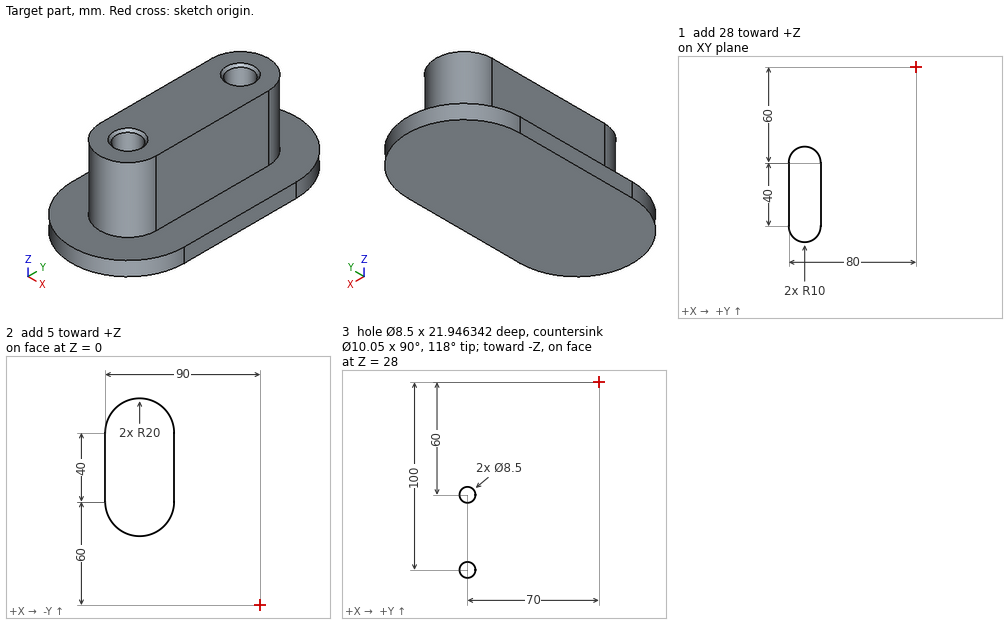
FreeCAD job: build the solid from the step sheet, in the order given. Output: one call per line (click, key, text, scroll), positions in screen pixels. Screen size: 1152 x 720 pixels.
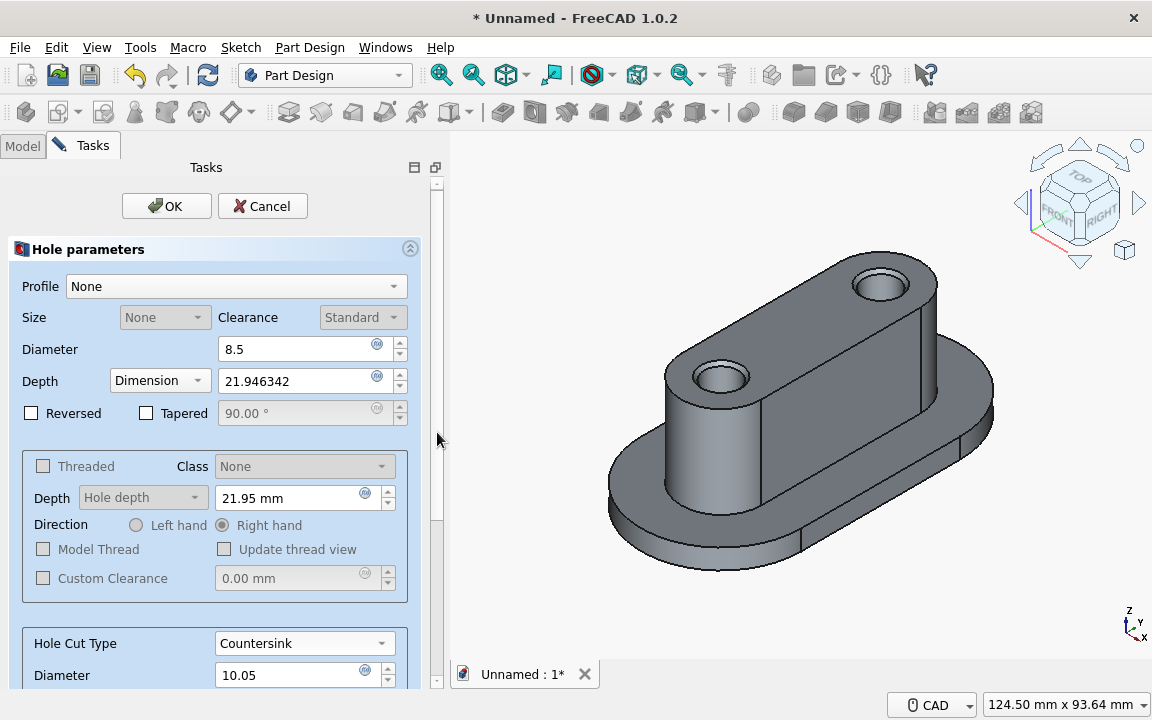
click(167, 206)